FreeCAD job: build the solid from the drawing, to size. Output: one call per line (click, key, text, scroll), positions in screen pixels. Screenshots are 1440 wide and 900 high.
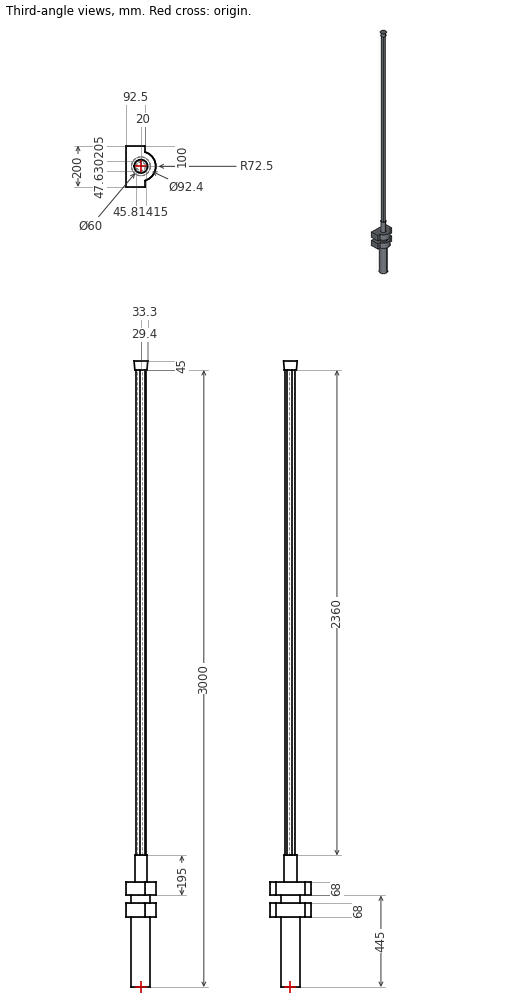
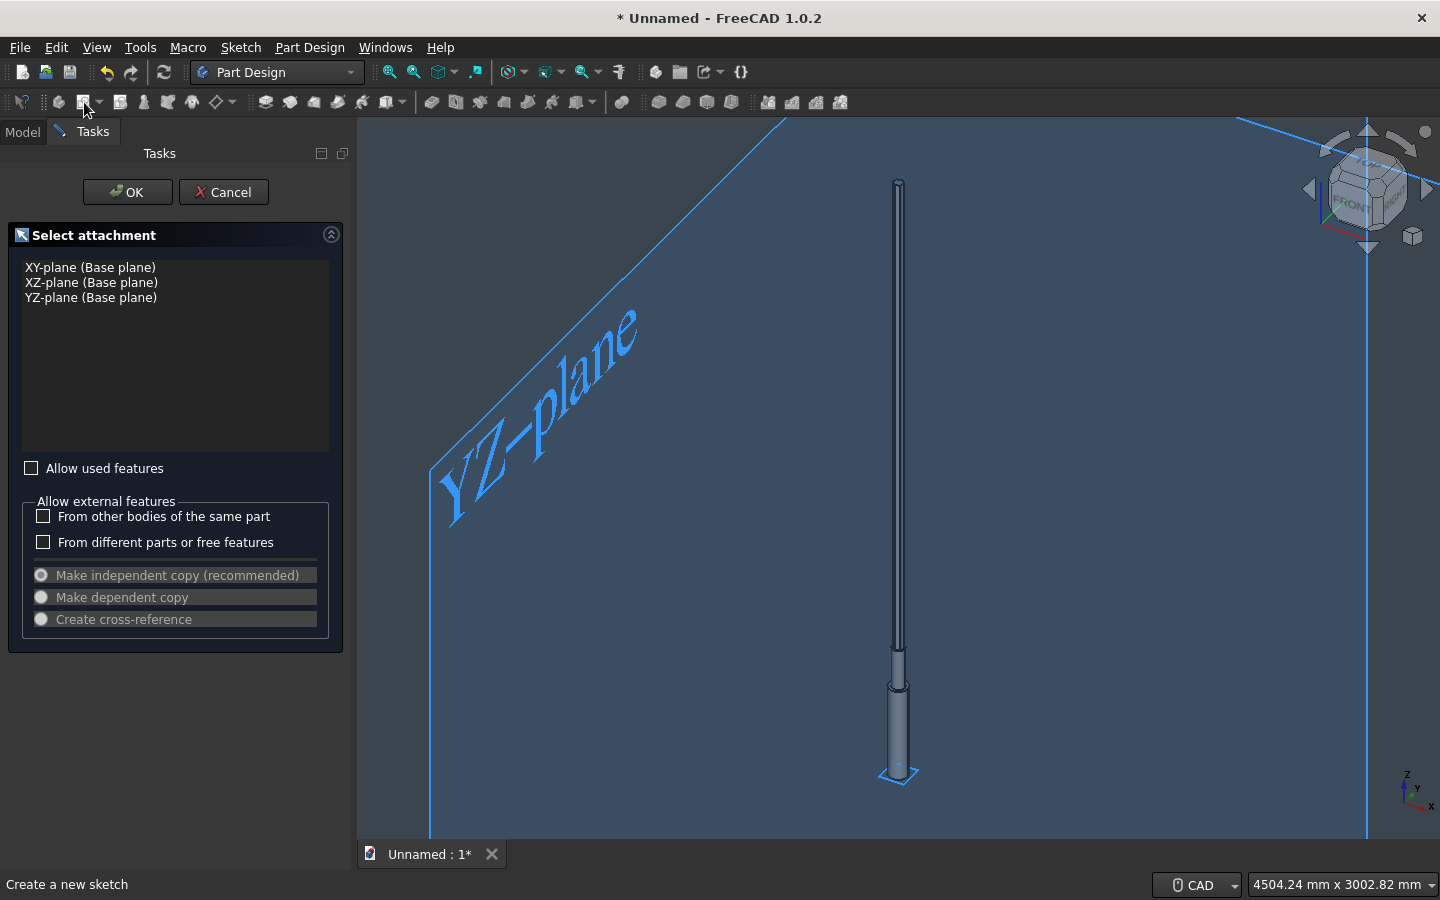
click(82, 282)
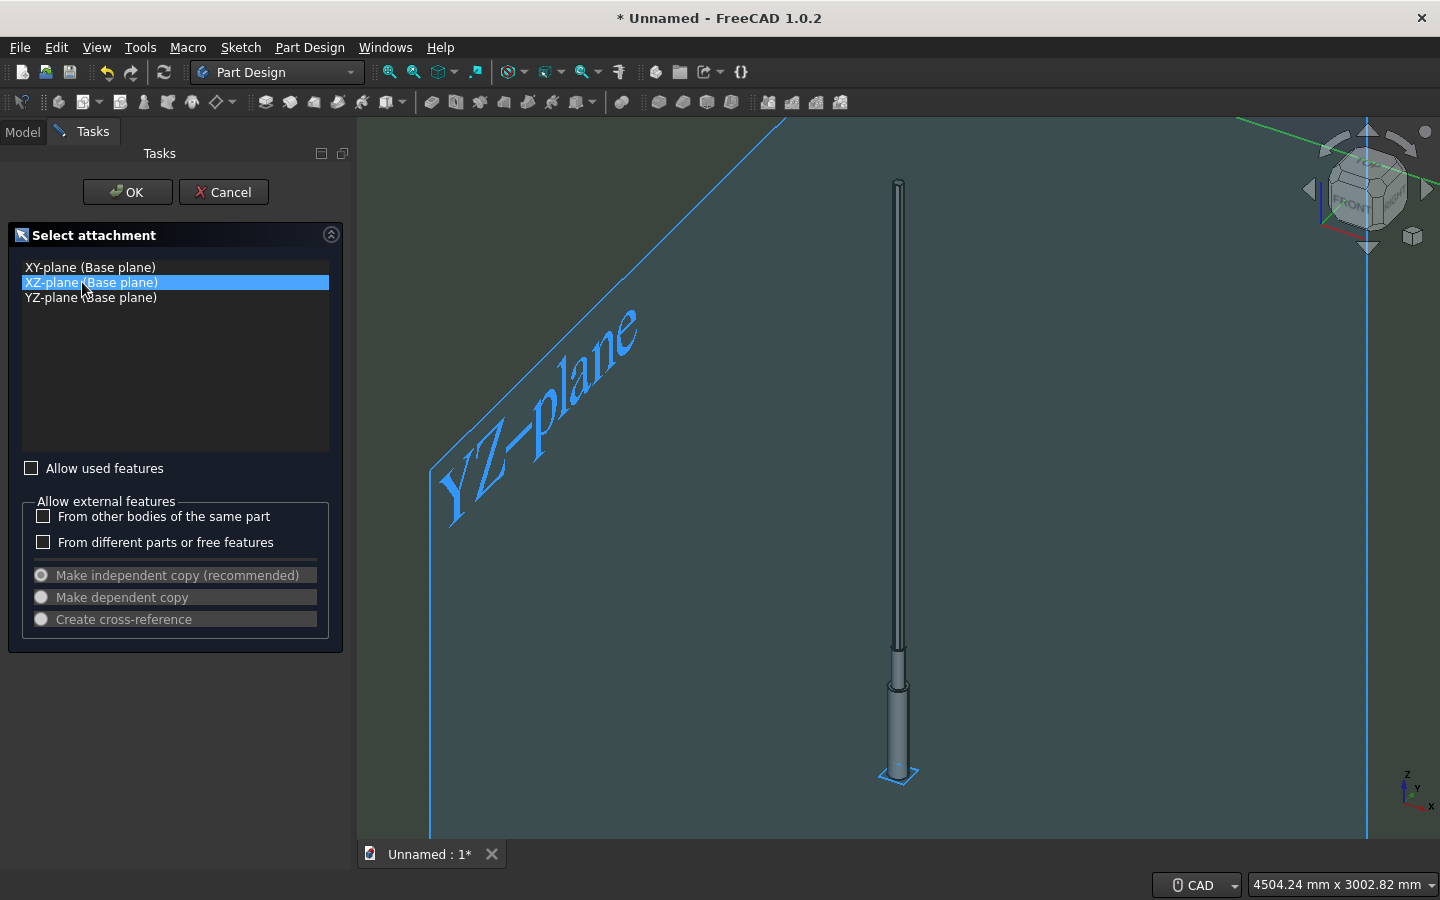
click(128, 192)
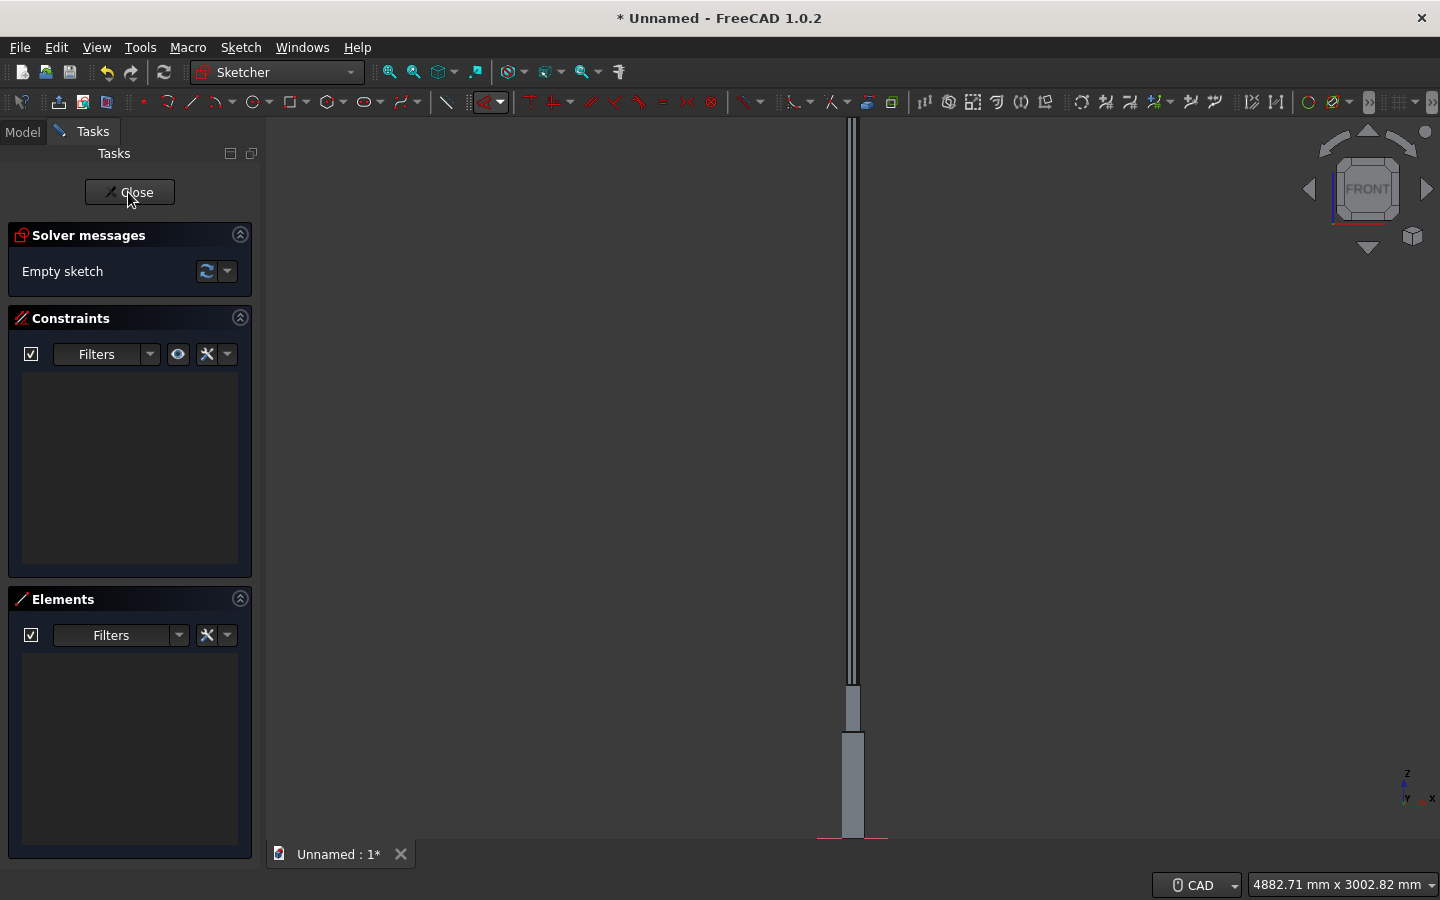
key(q)
key(s)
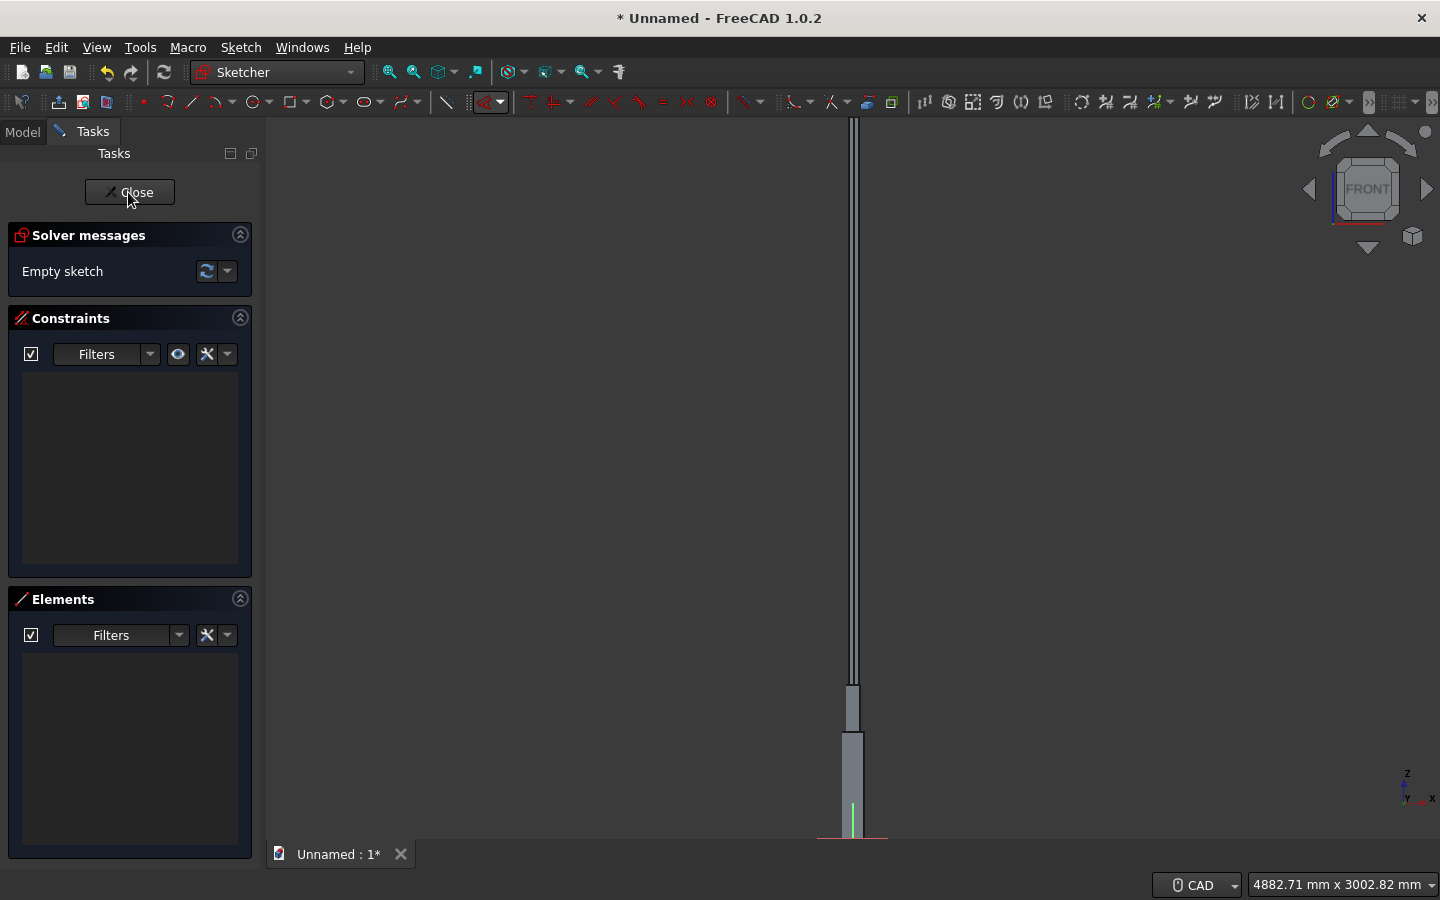
scroll(784, 478, down, 5)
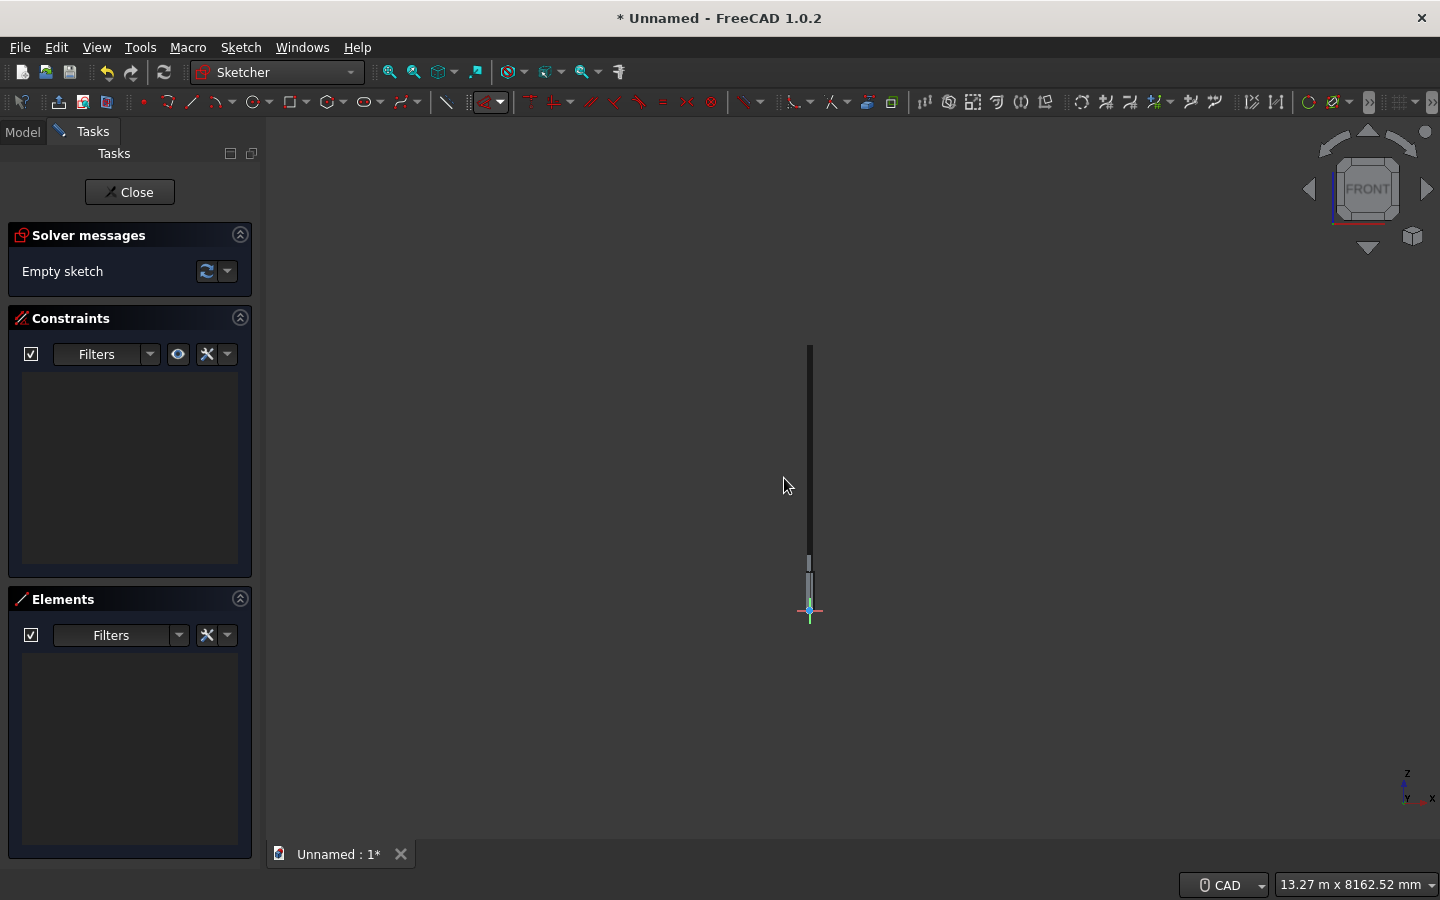
scroll(813, 337, up, 15)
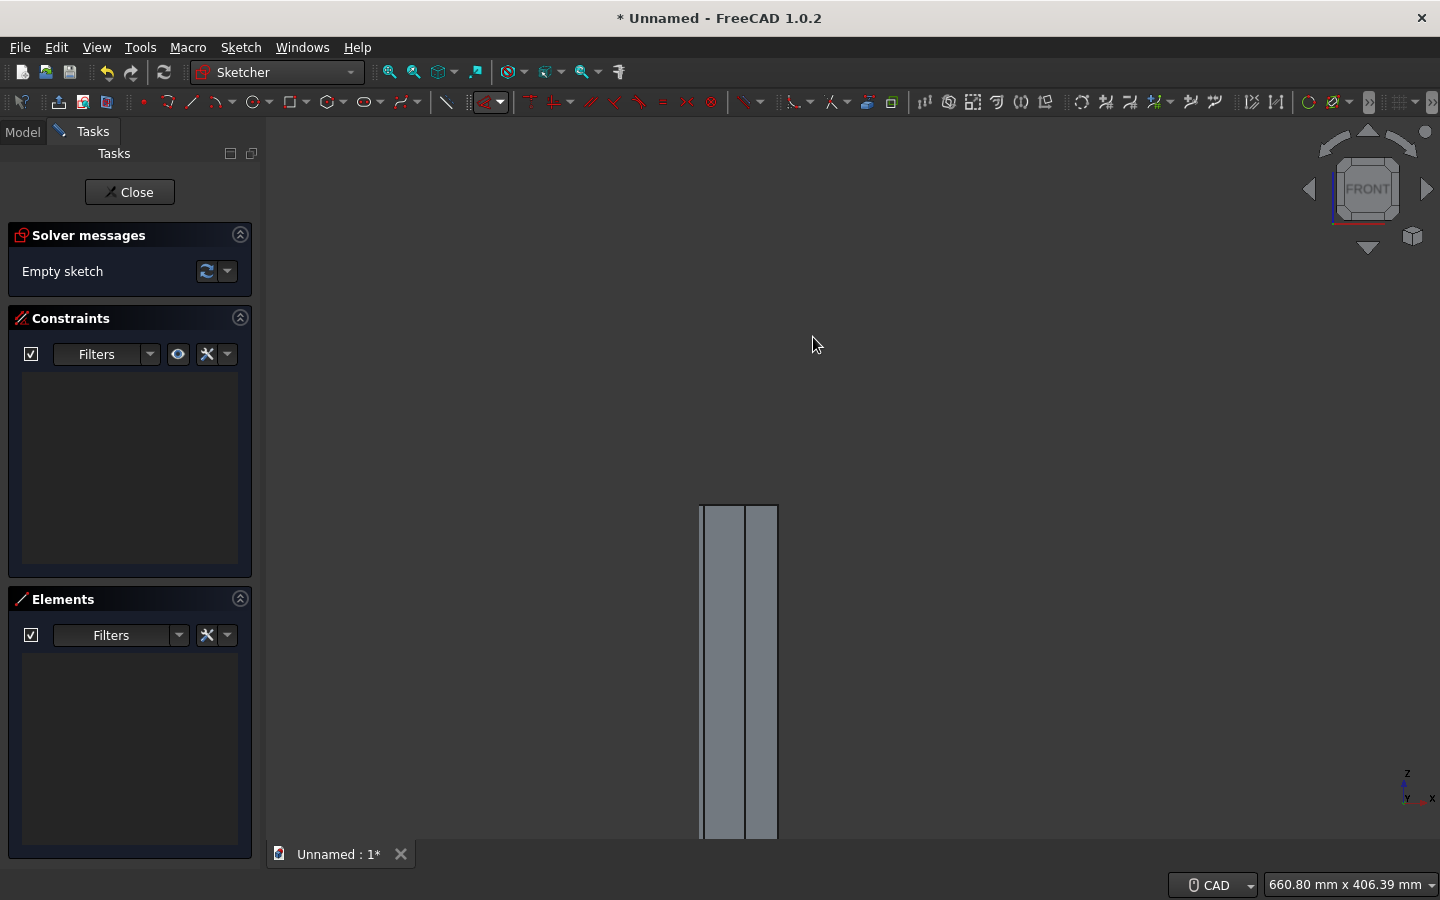
scroll(763, 462, up, 9)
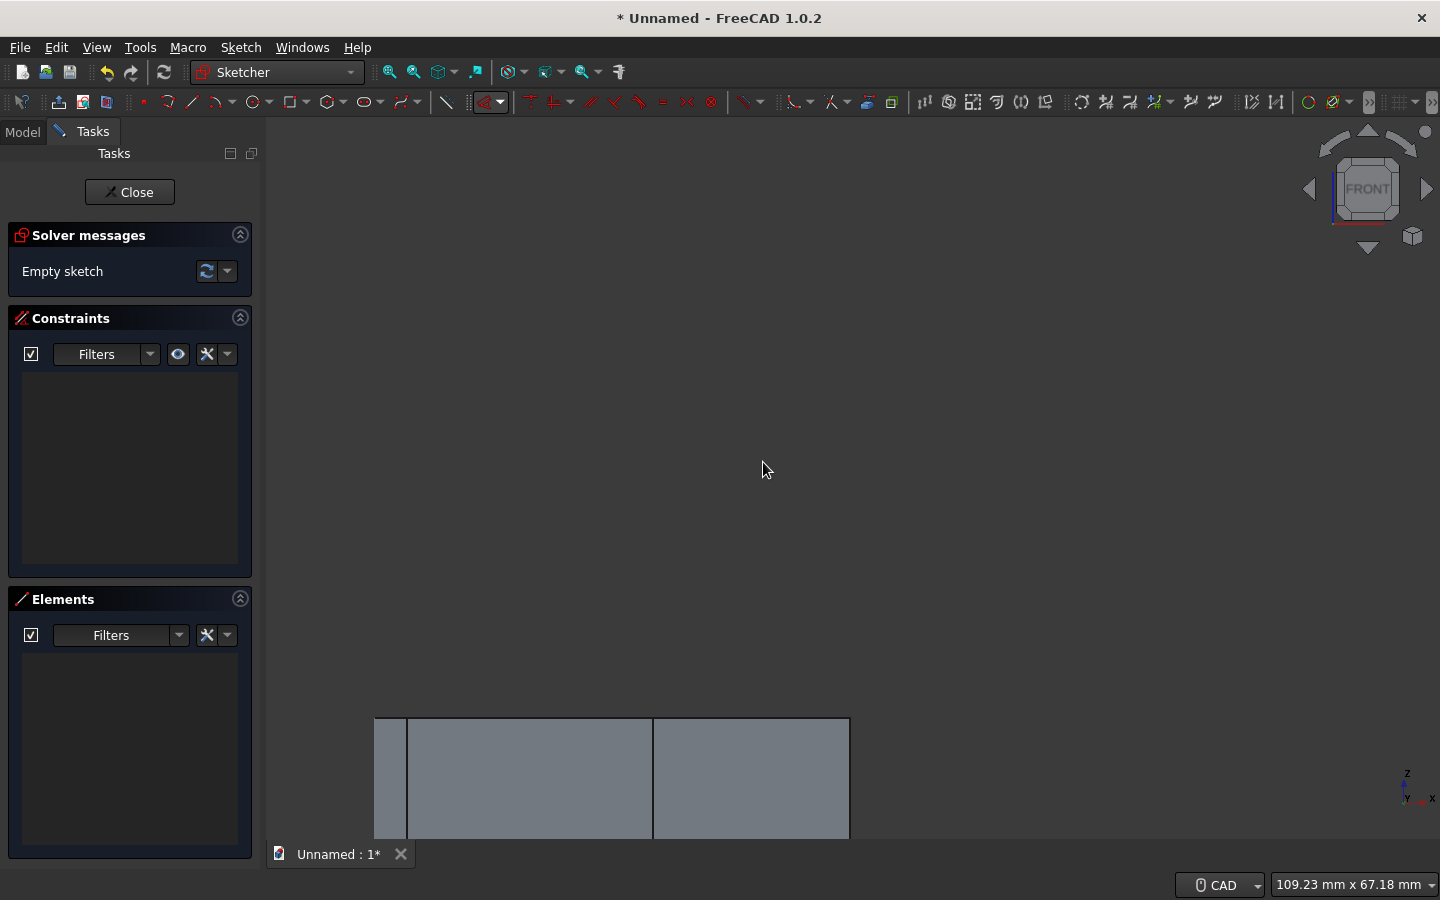
key(g)
key(m)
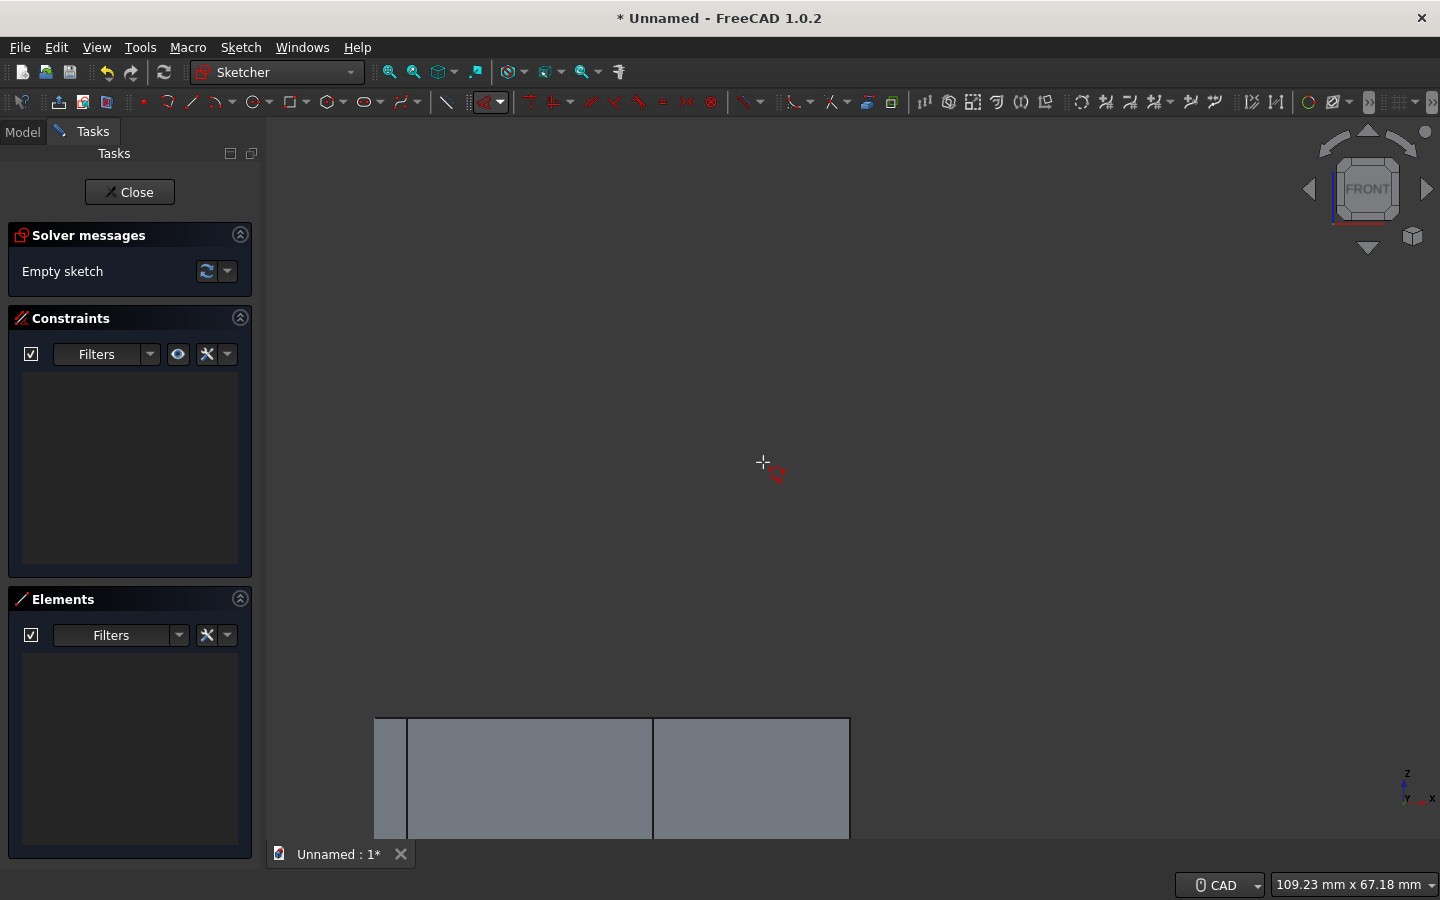
click(604, 718)
click(613, 234)
click(962, 234)
click(920, 718)
click(604, 719)
key(Escape)
key(Escape)